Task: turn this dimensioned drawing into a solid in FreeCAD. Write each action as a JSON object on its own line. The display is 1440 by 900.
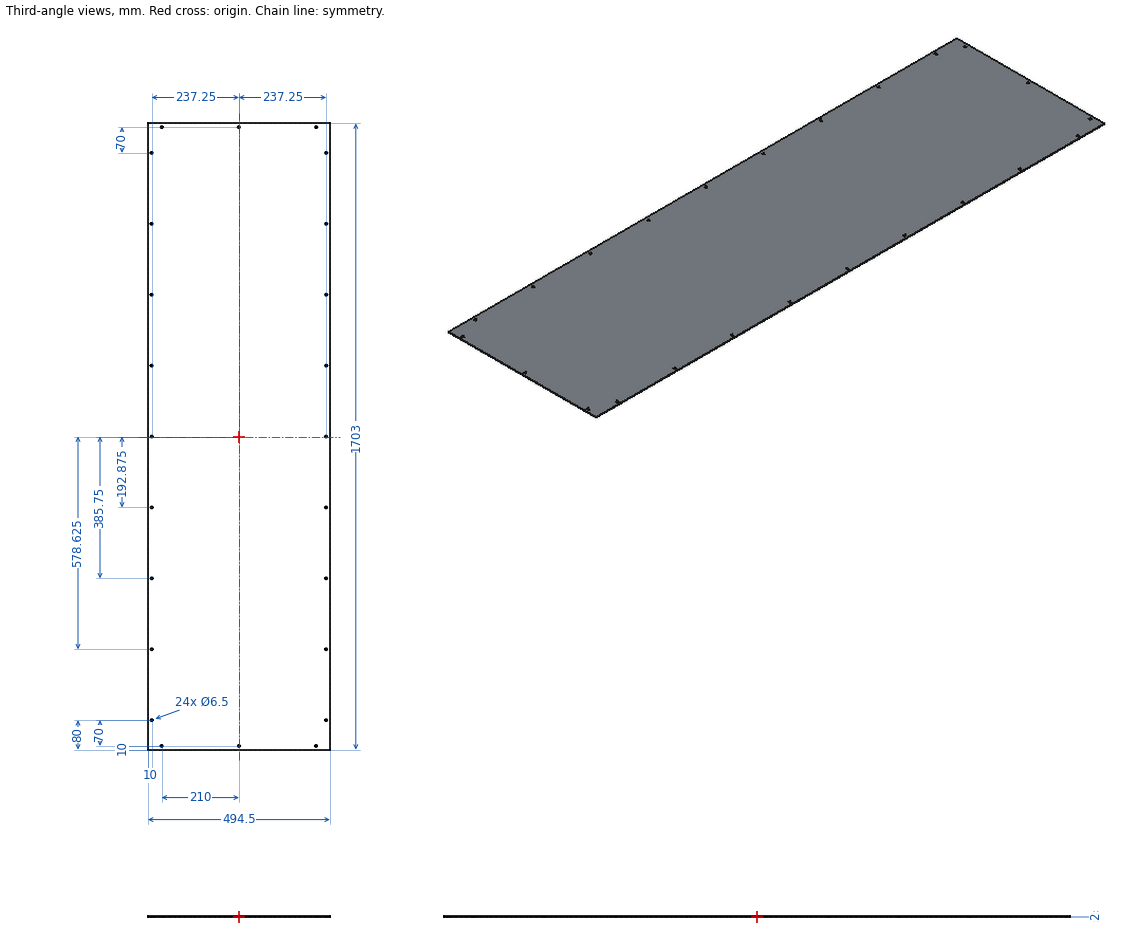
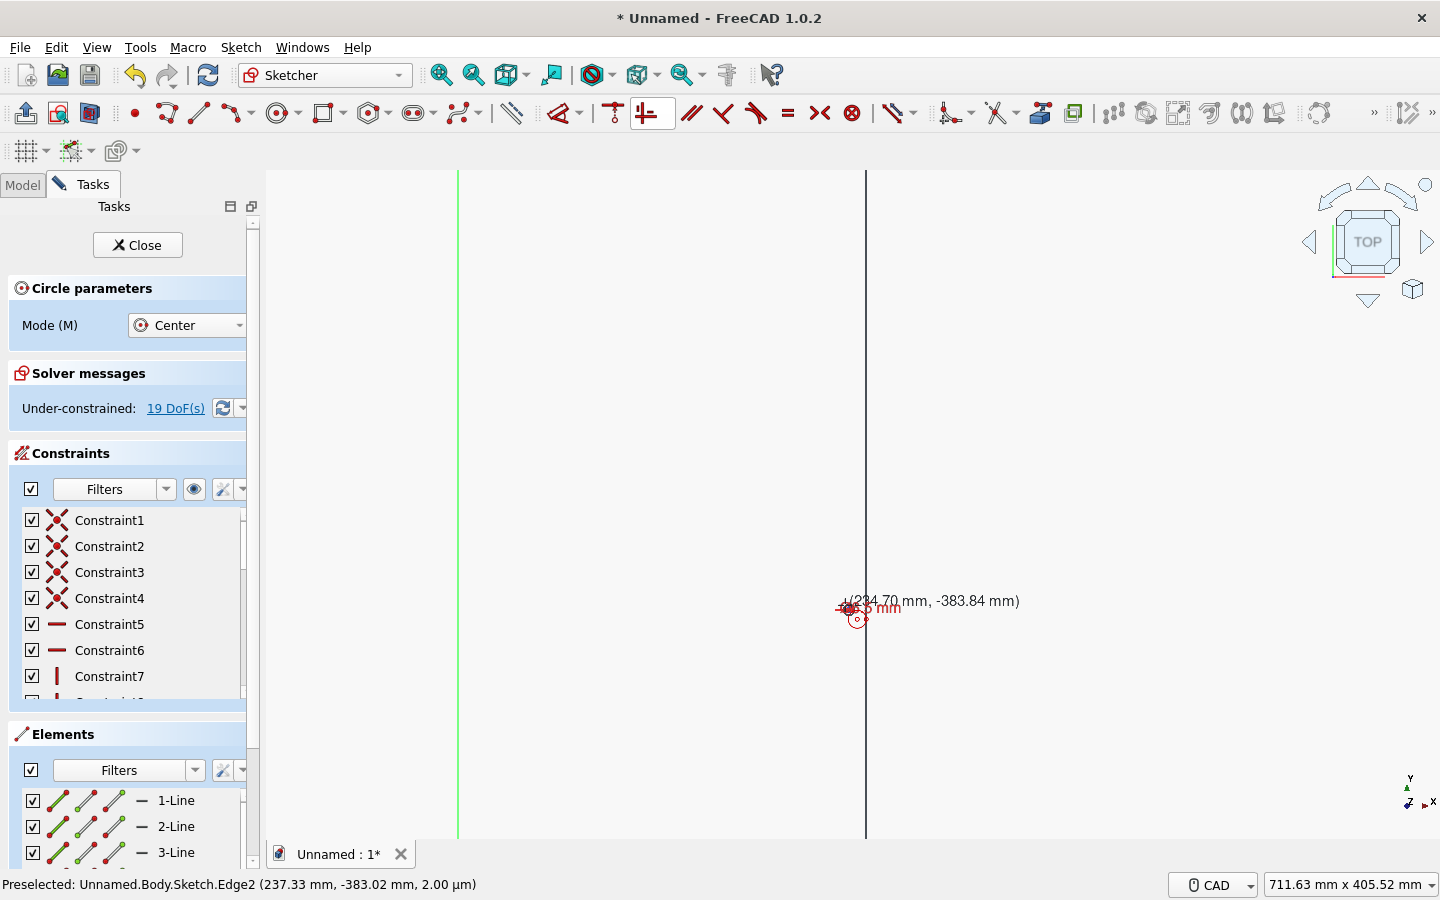
{"action": "scroll", "coordinate": [849, 291], "scroll_direction": "up", "scroll_amount": 8}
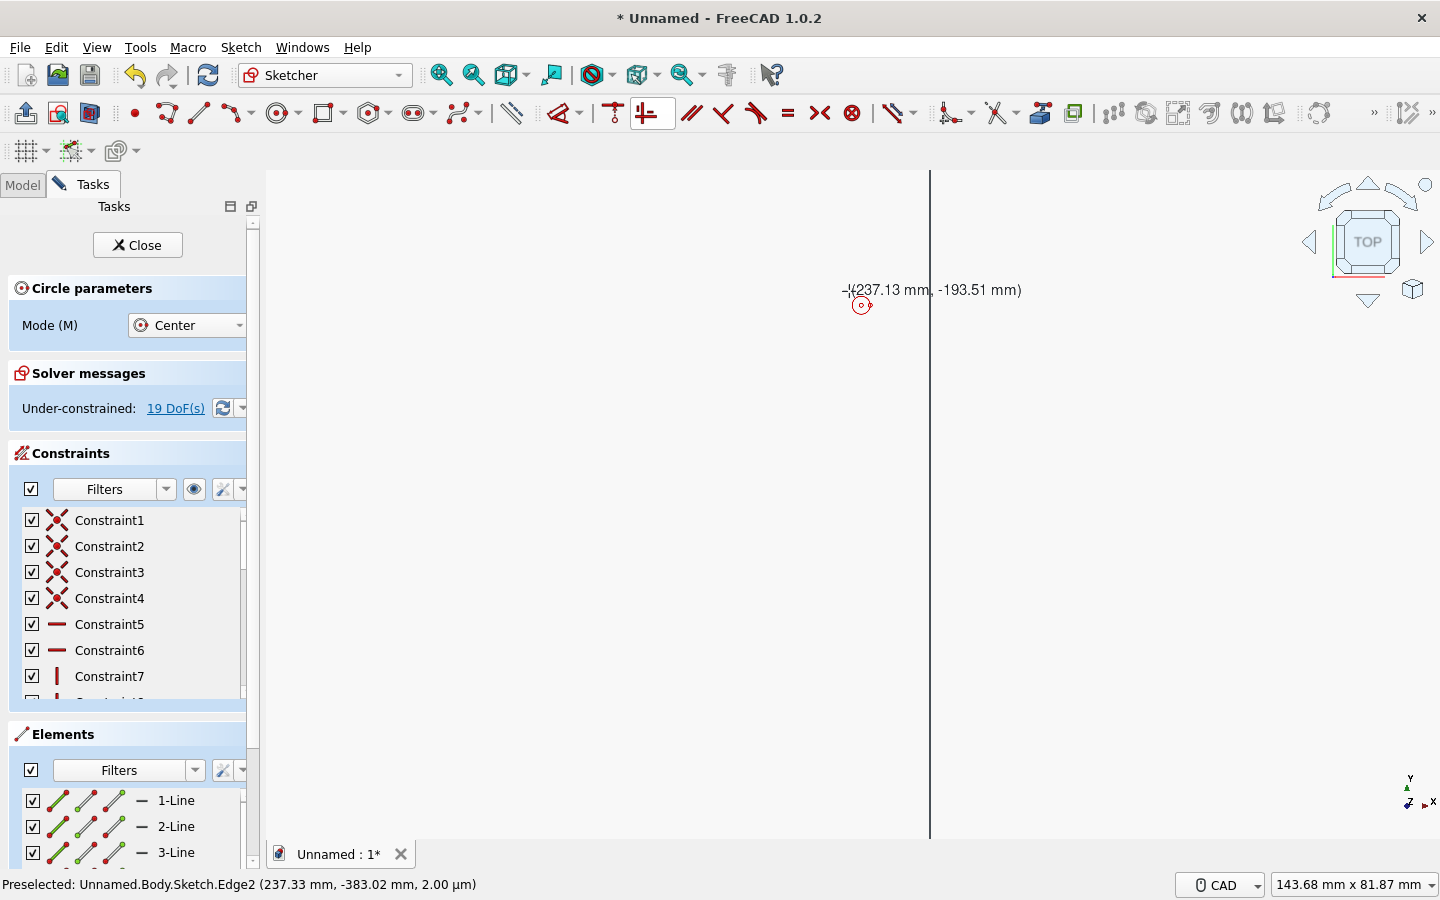
{"action": "scroll", "coordinate": [849, 566], "scroll_direction": "down", "scroll_amount": 17}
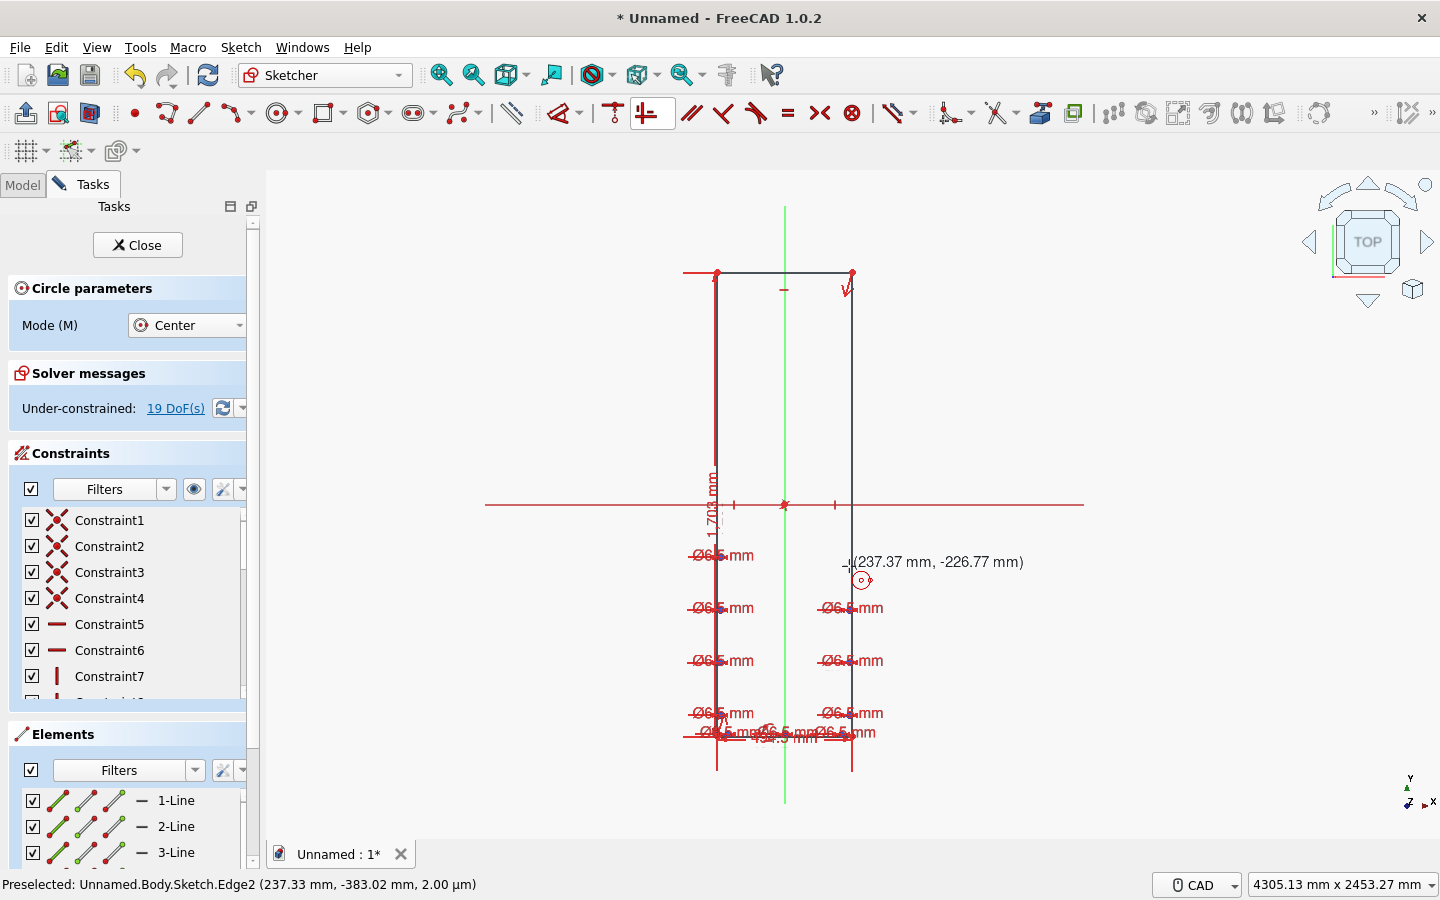
{"action": "scroll", "coordinate": [849, 557], "scroll_direction": "up", "scroll_amount": 9}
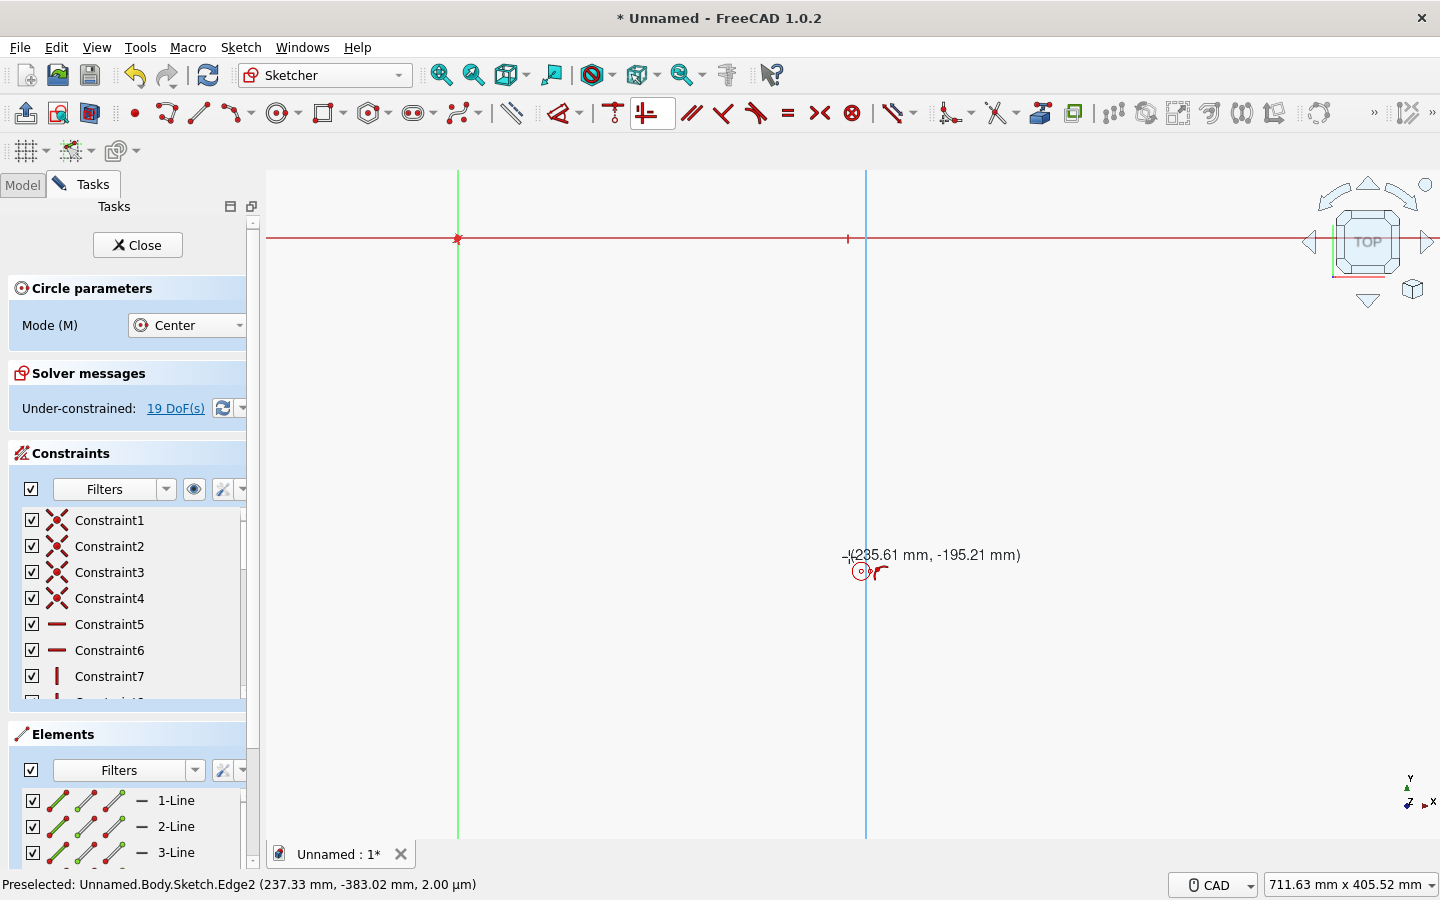
{"action": "left_click", "coordinate": [849, 556]}
{"action": "mouse_move", "coordinate": [845, 552]}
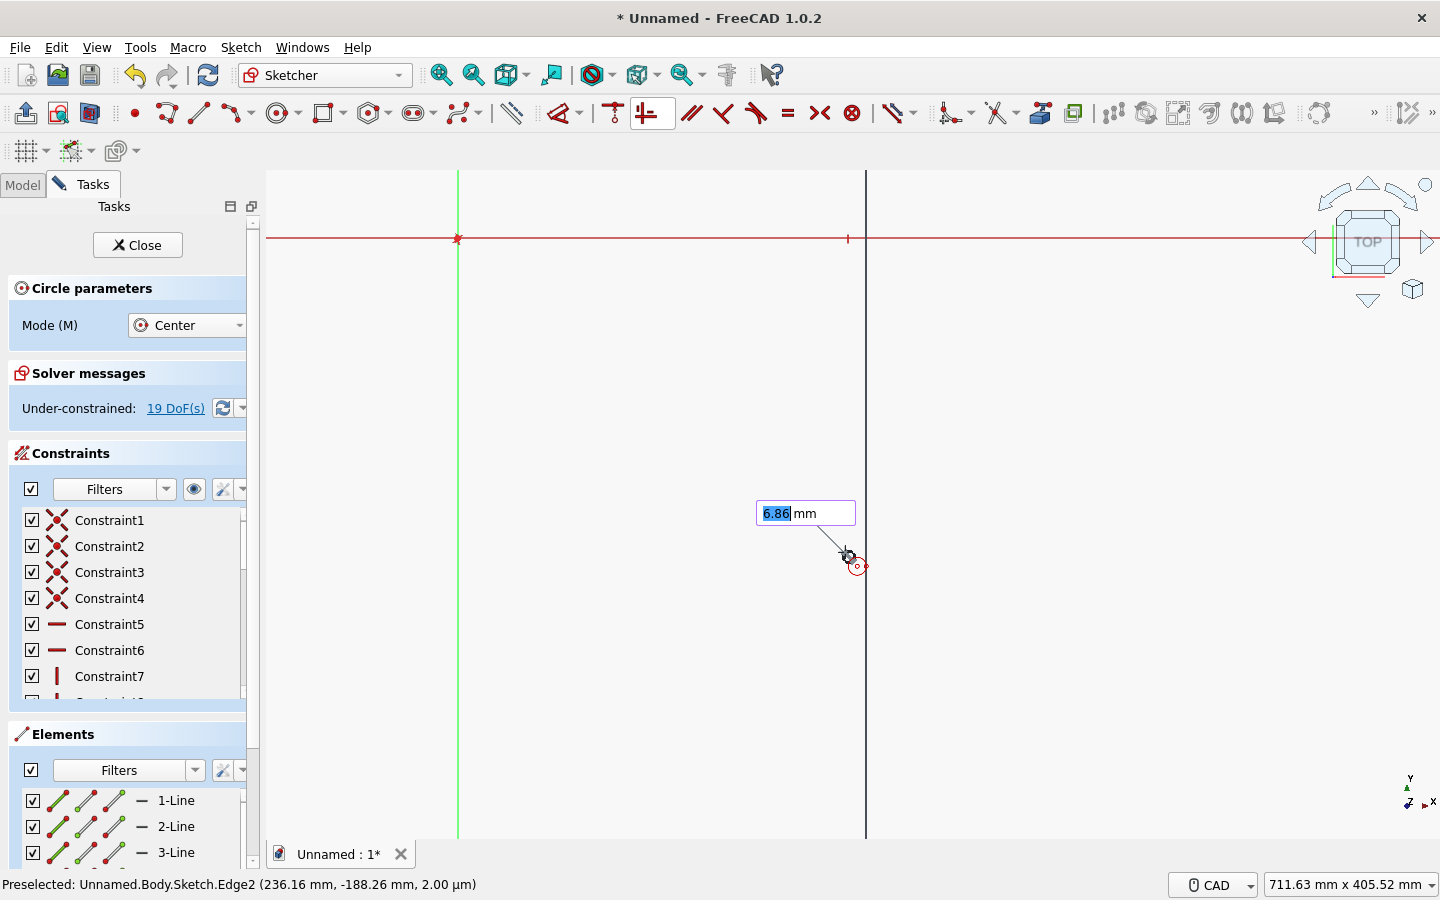
{"action": "type", "text": "6.5"}
{"action": "key", "text": "Return"}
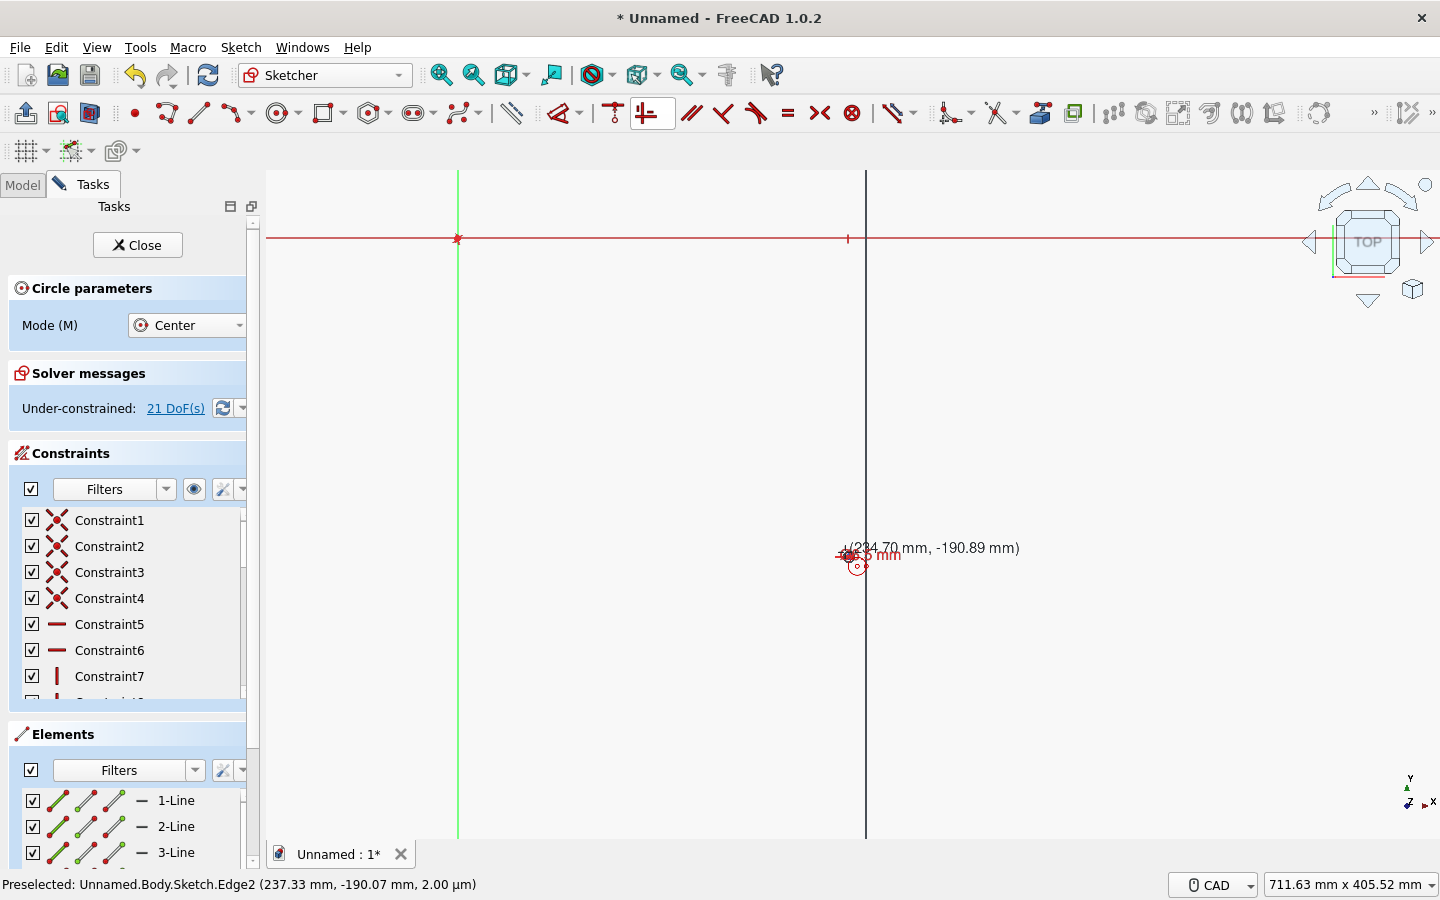
{"action": "scroll", "coordinate": [849, 557], "scroll_direction": "down", "scroll_amount": 9}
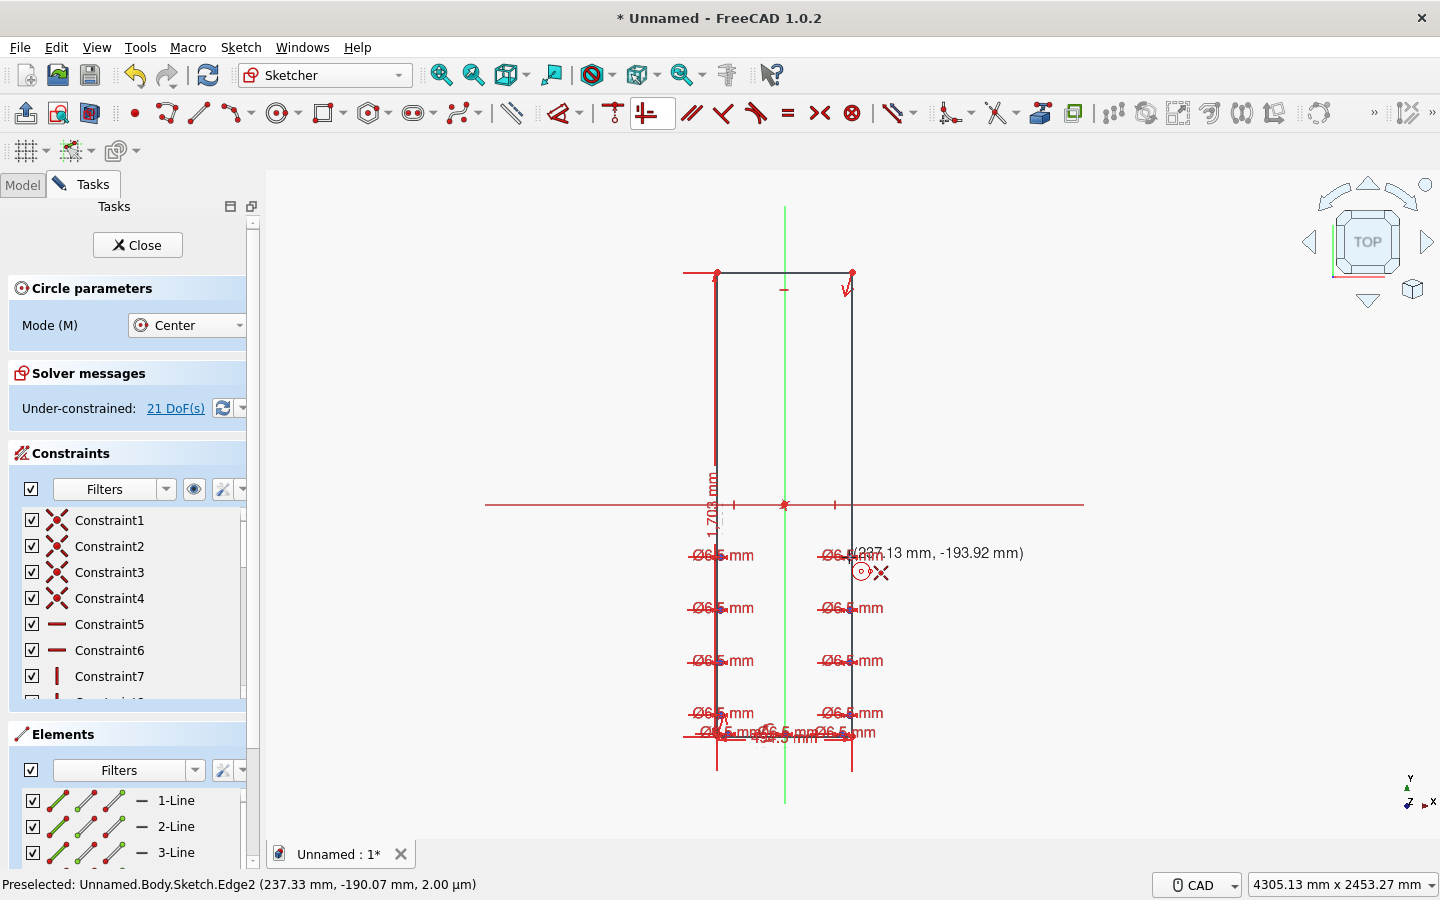
{"action": "scroll", "coordinate": [720, 505], "scroll_direction": "up", "scroll_amount": 17}